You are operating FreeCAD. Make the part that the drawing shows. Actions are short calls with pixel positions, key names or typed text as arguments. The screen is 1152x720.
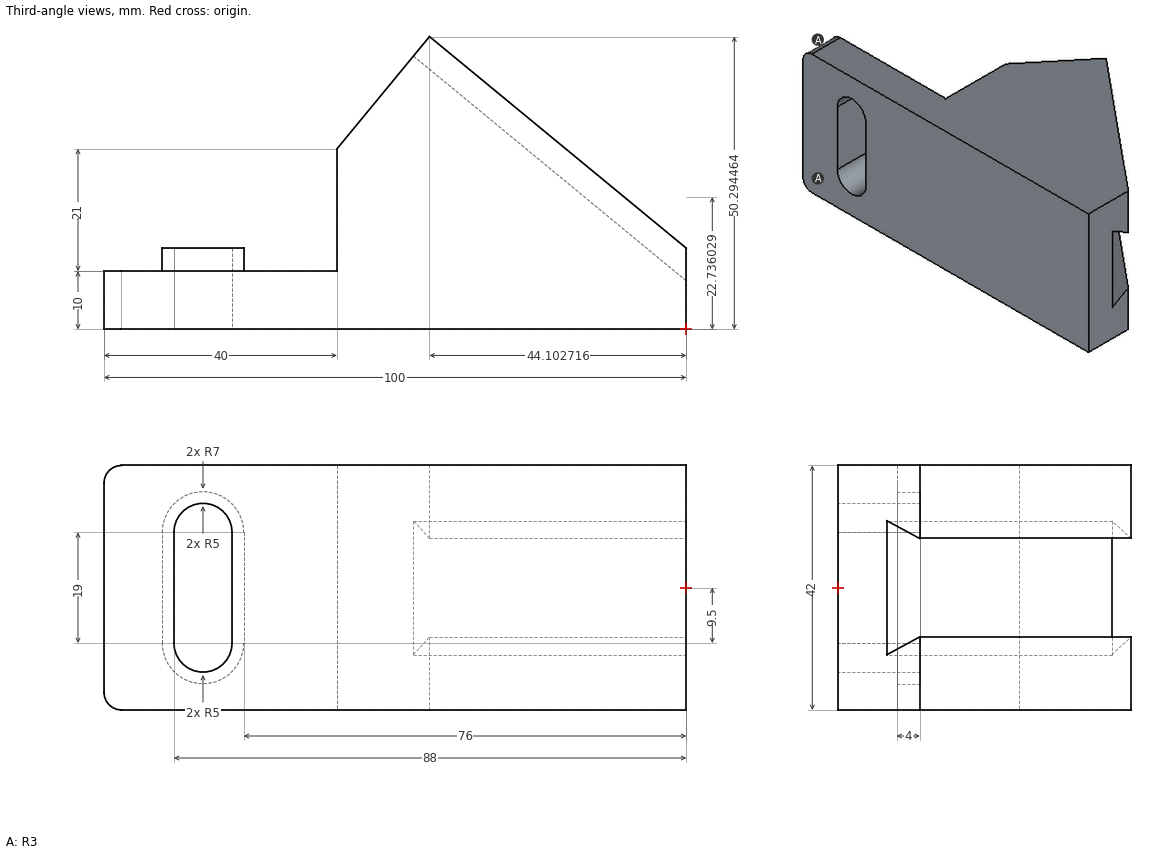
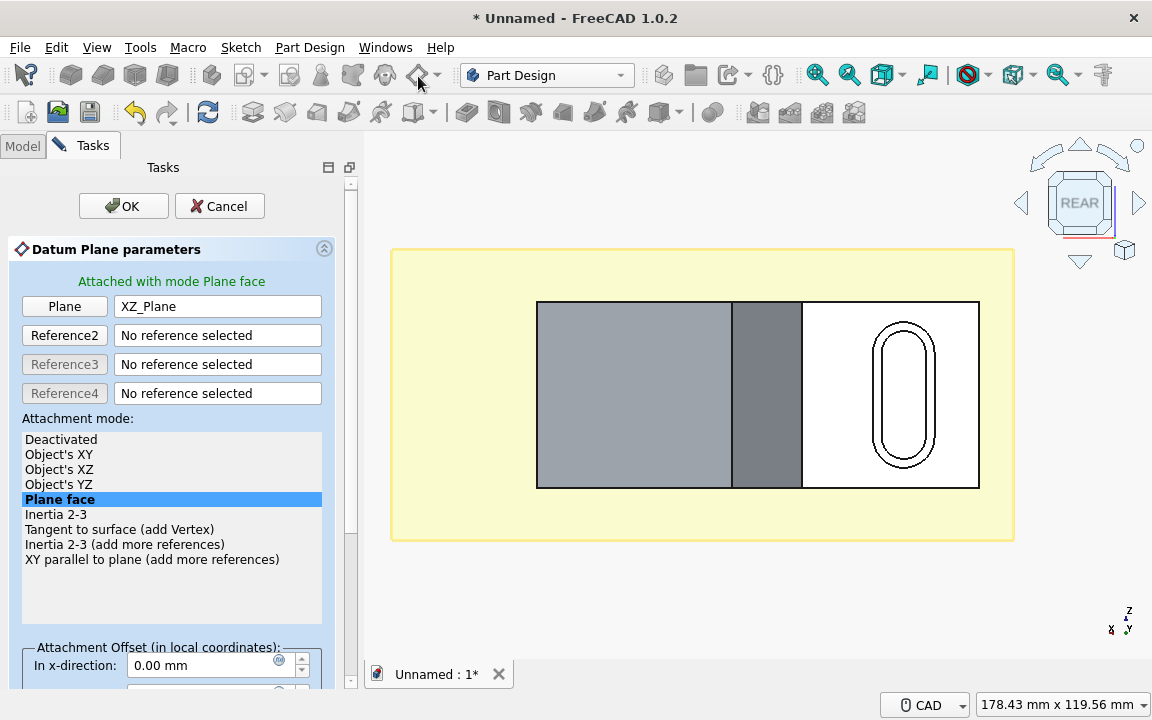
scroll(351, 432, down, 2)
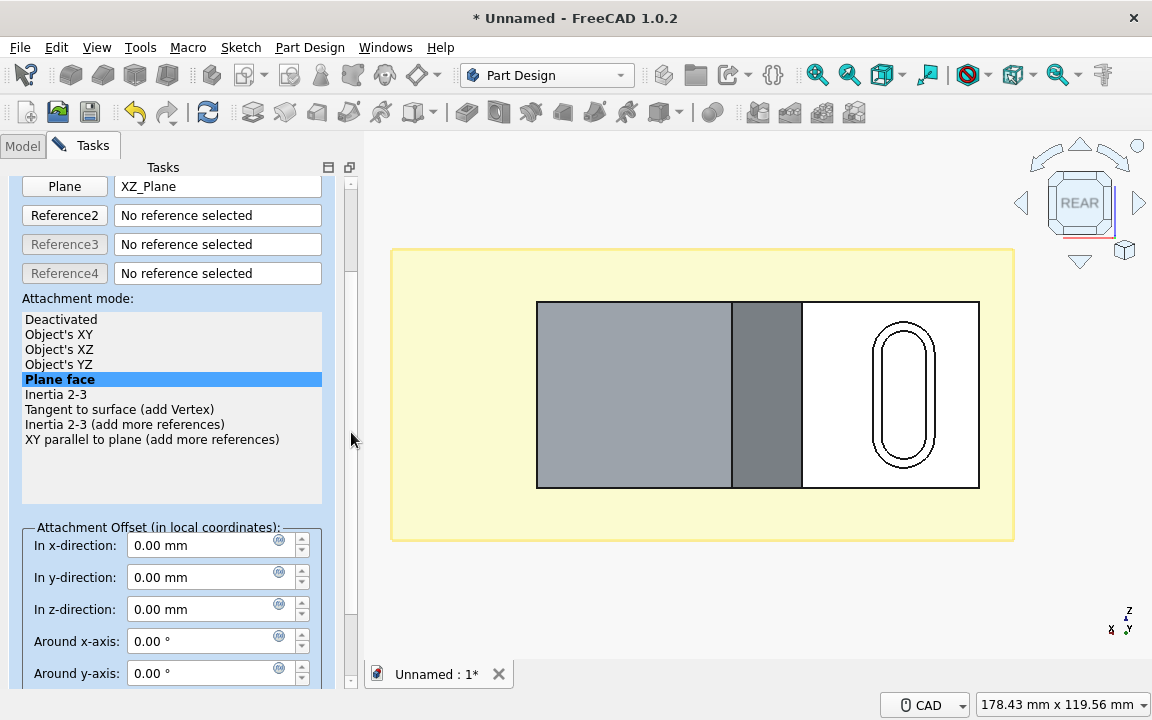
triple_click(210, 609)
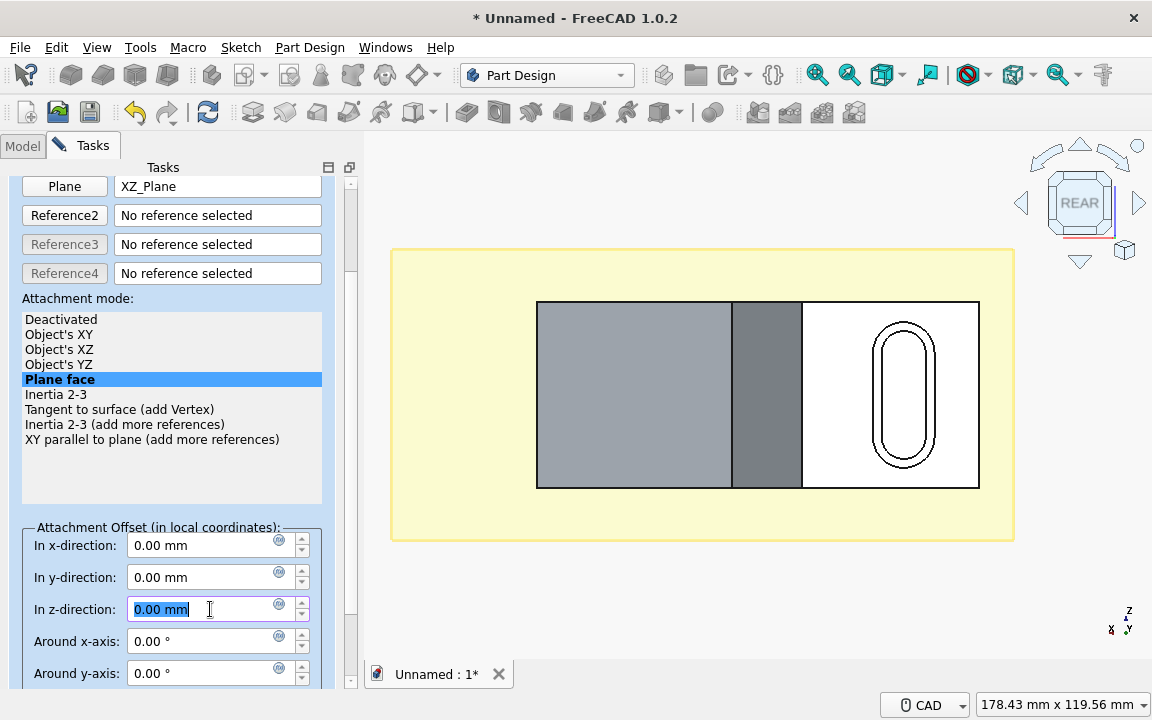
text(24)
key(Tab)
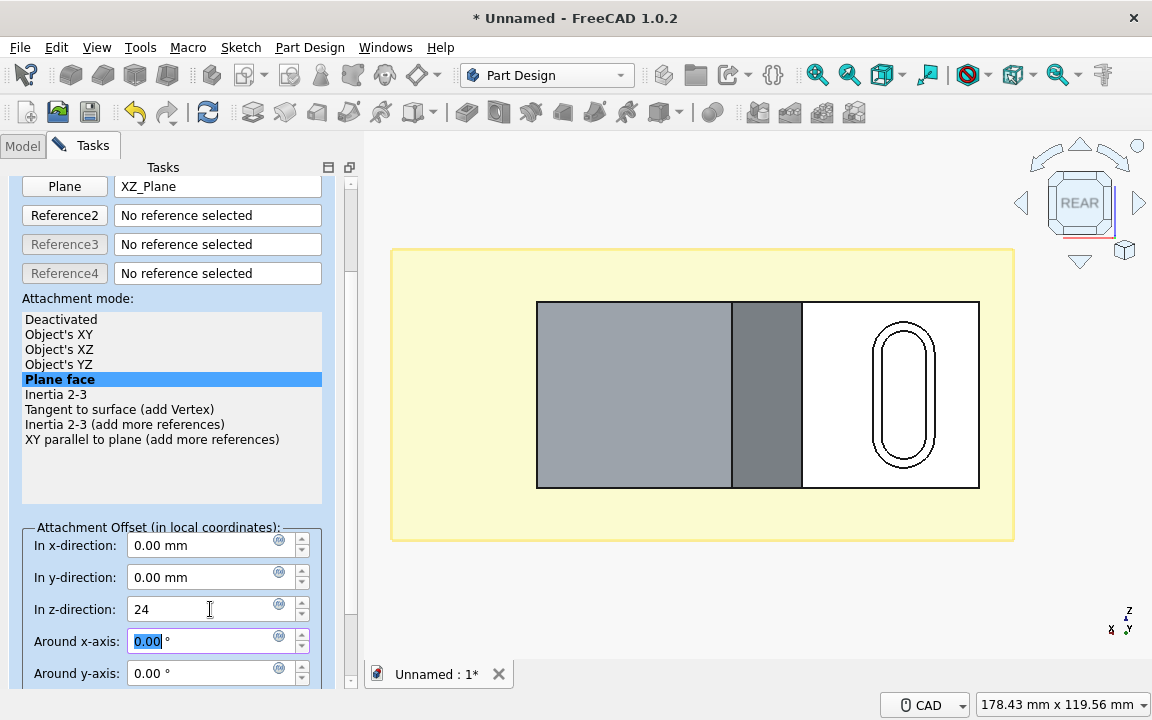
scroll(351, 432, up, 3)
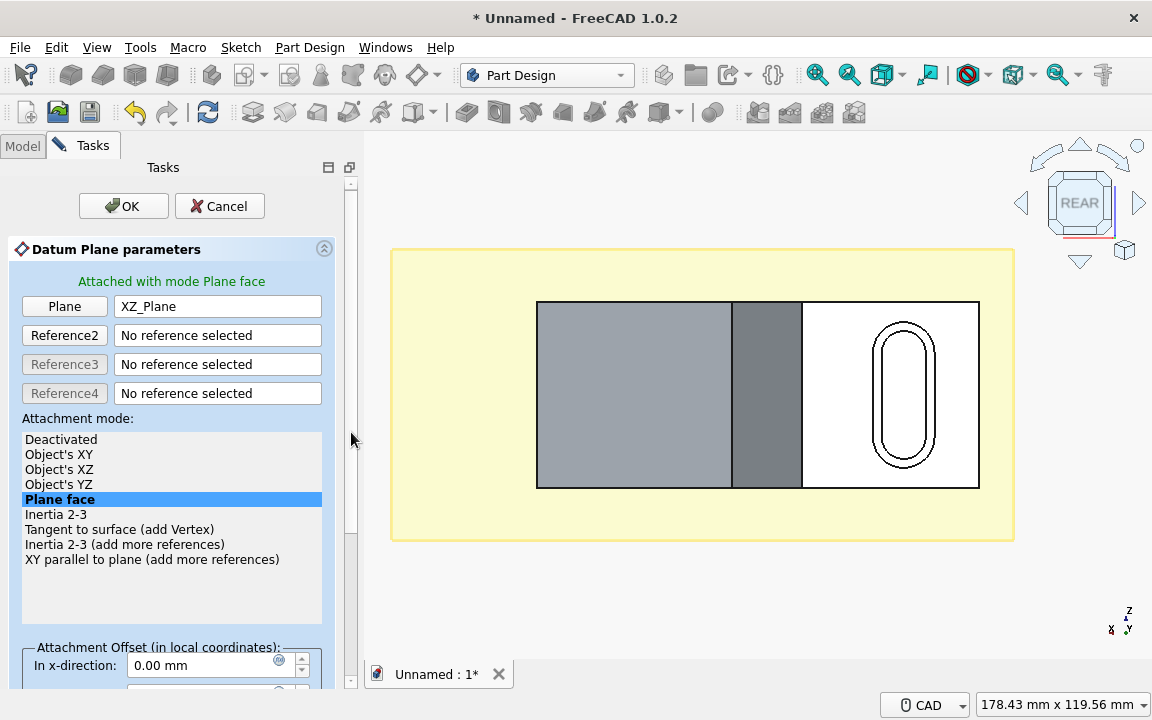
click(124, 206)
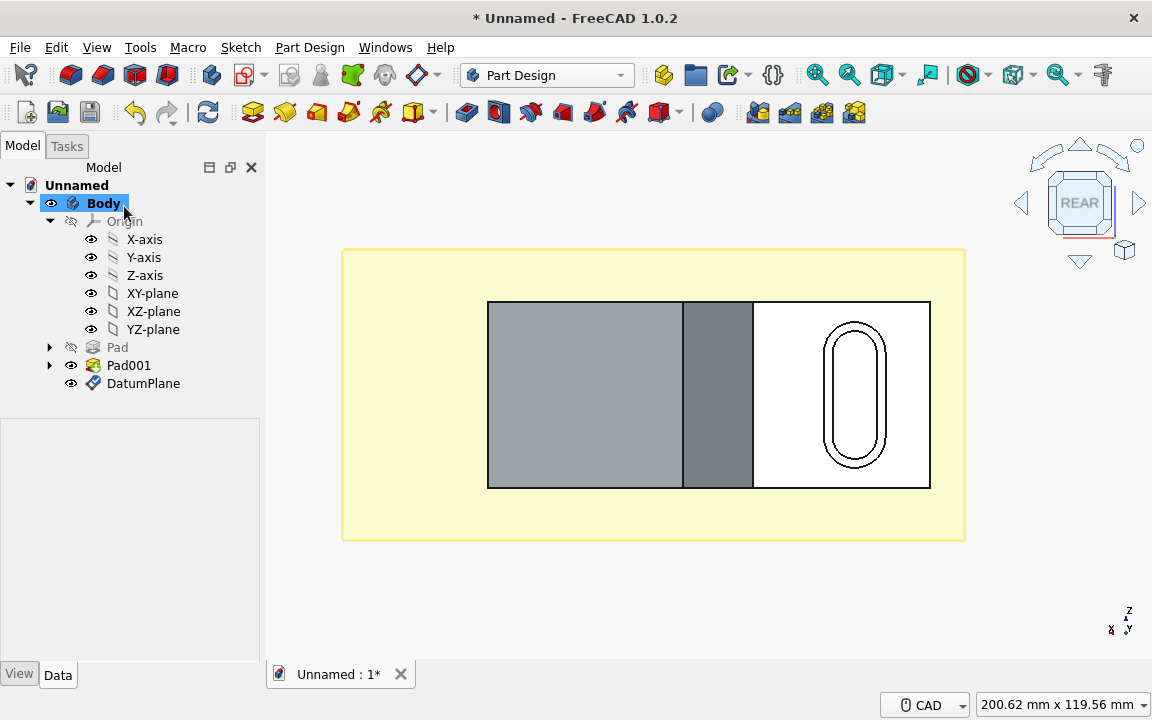
click(116, 383)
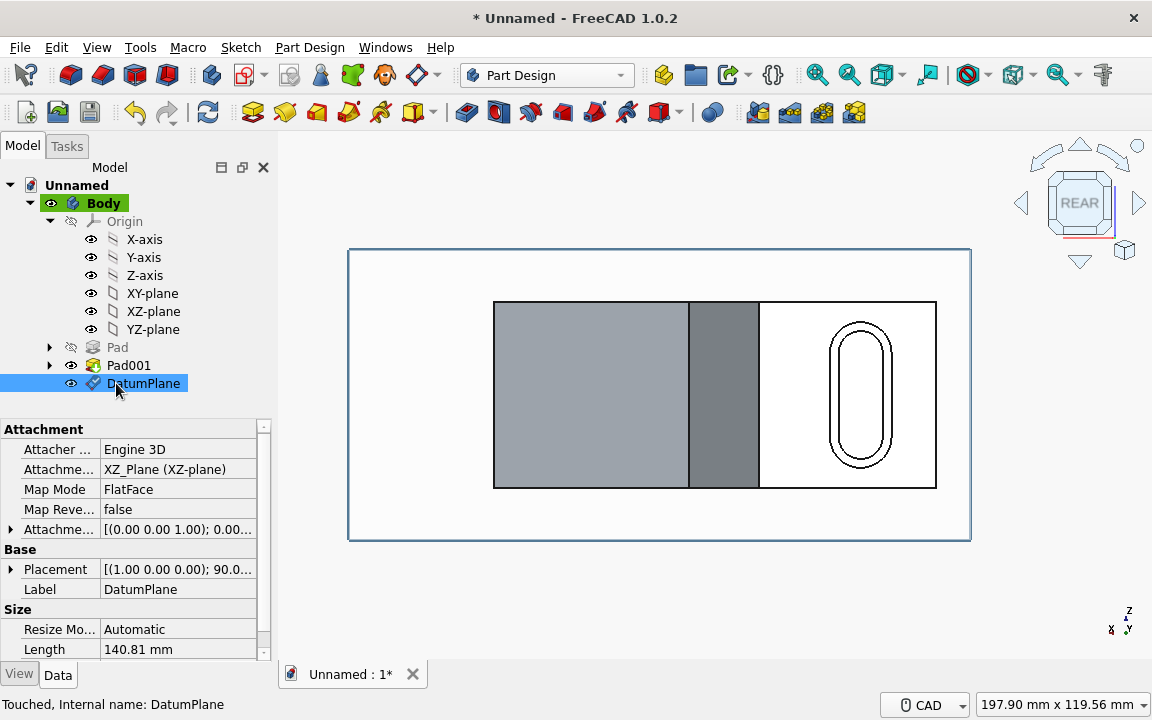
click(244, 76)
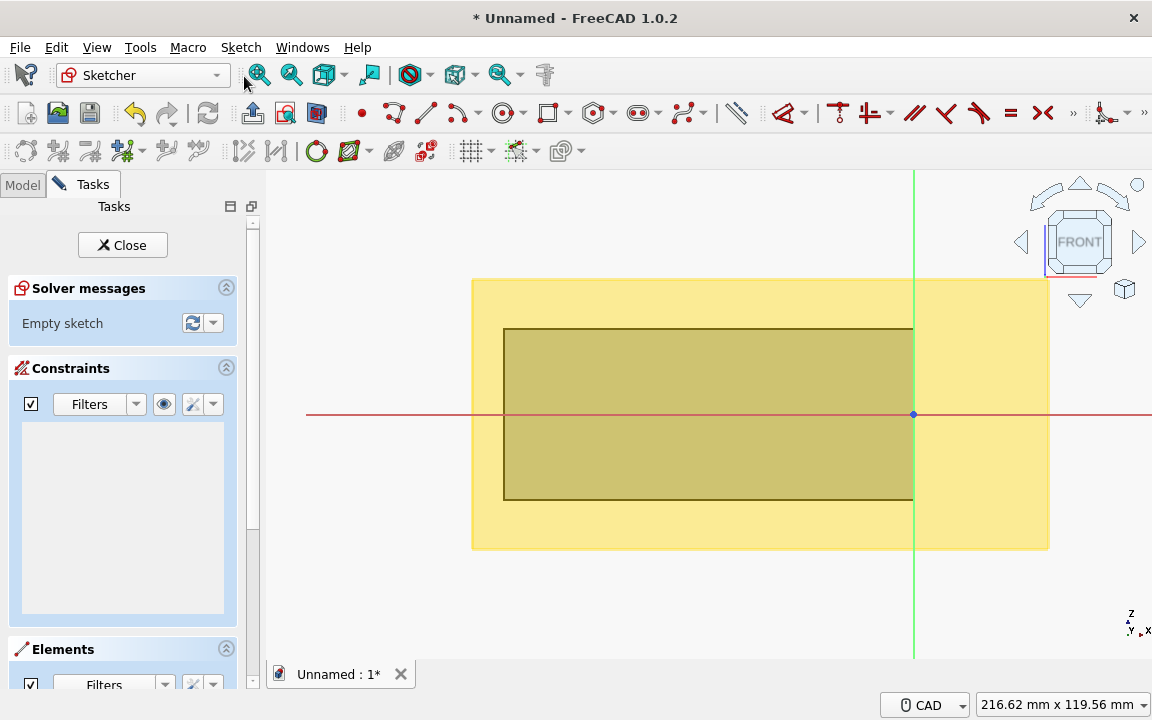
scroll(535, 415, up, 5)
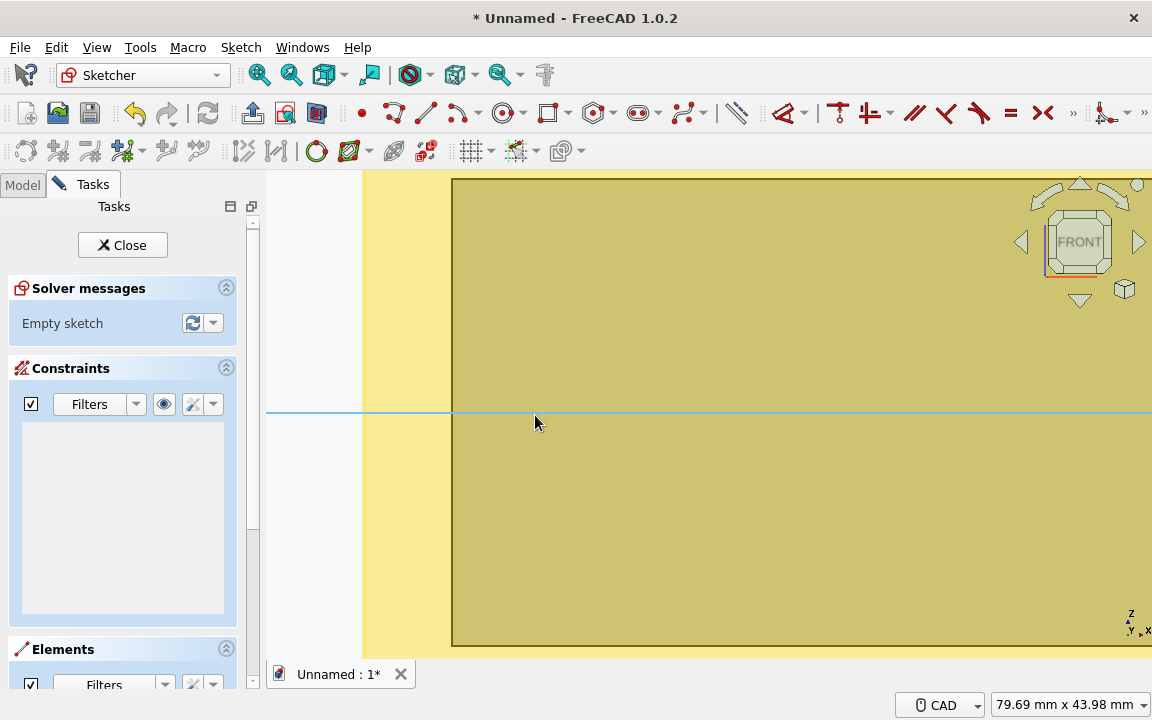
key(g)
key(s)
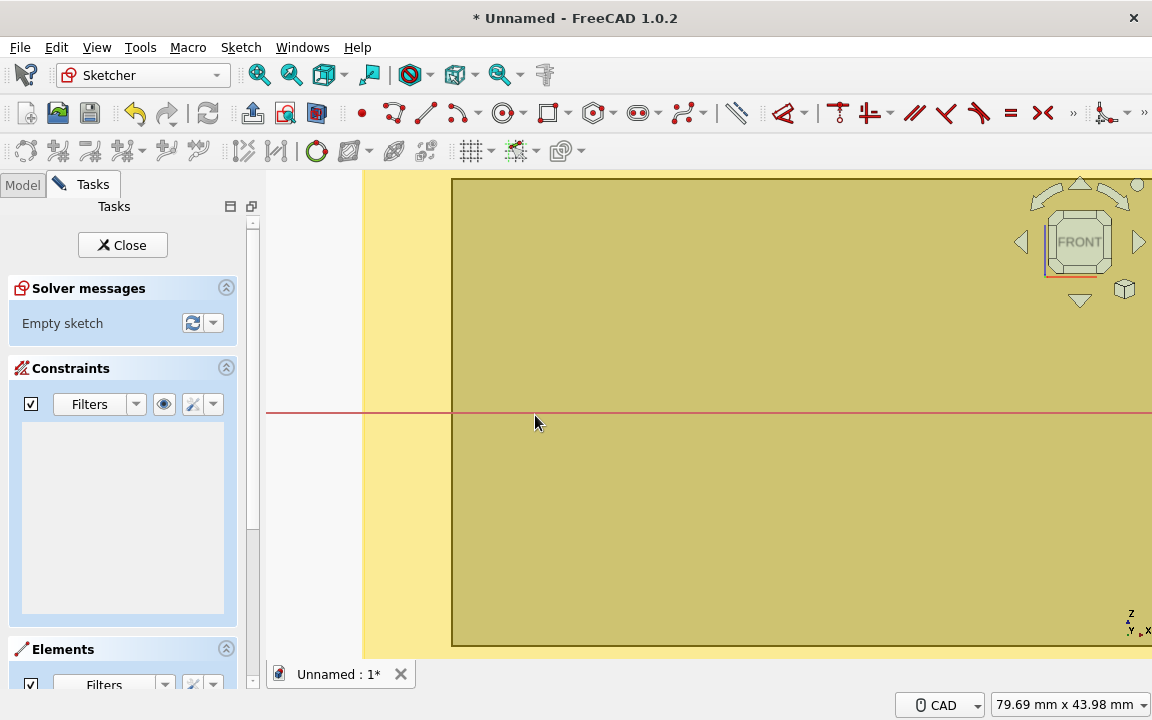
click(641, 518)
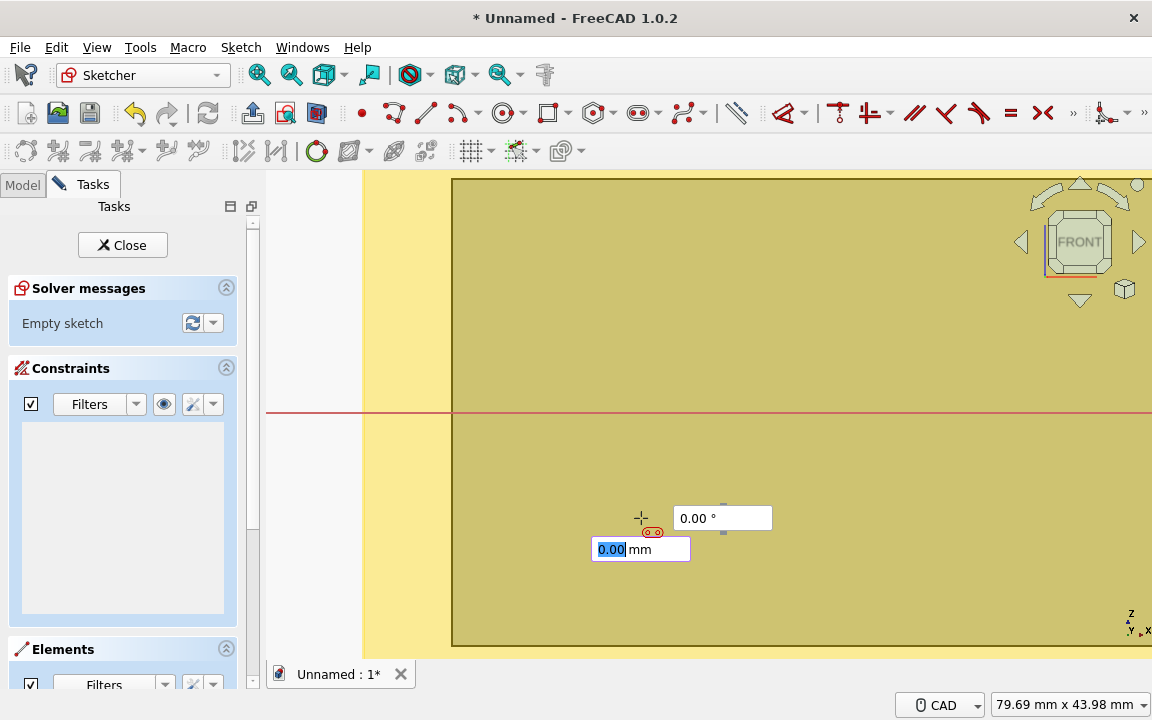
click(641, 307)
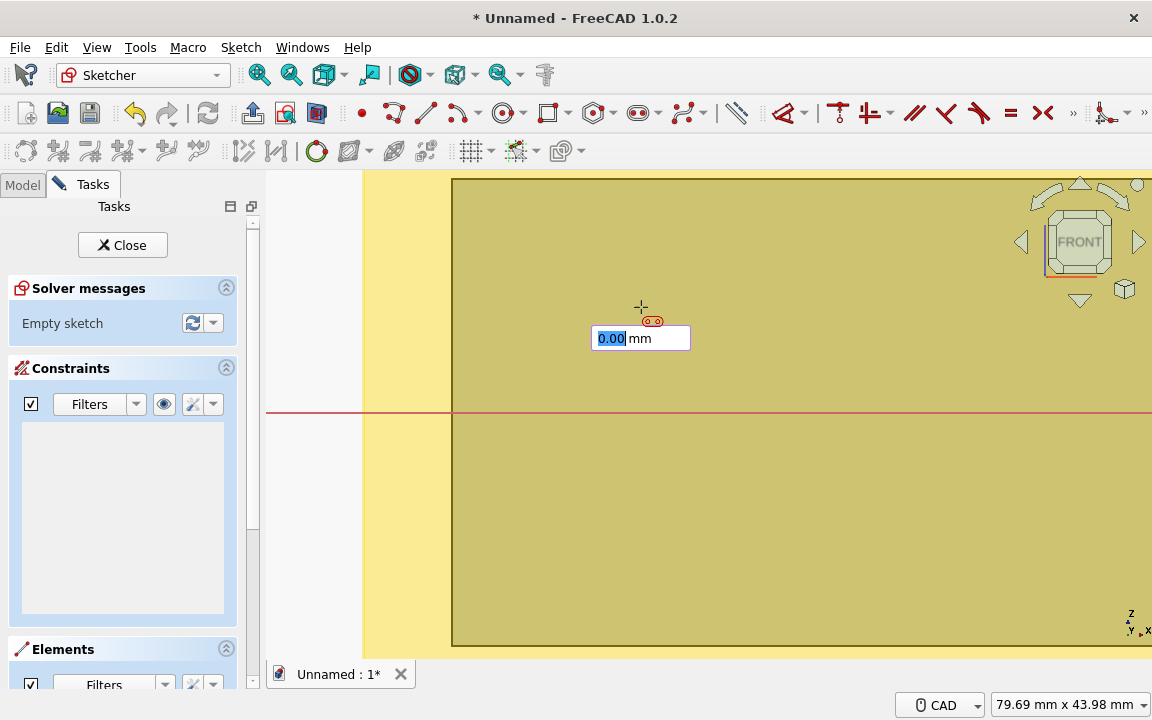
click(585, 444)
key(Escape)